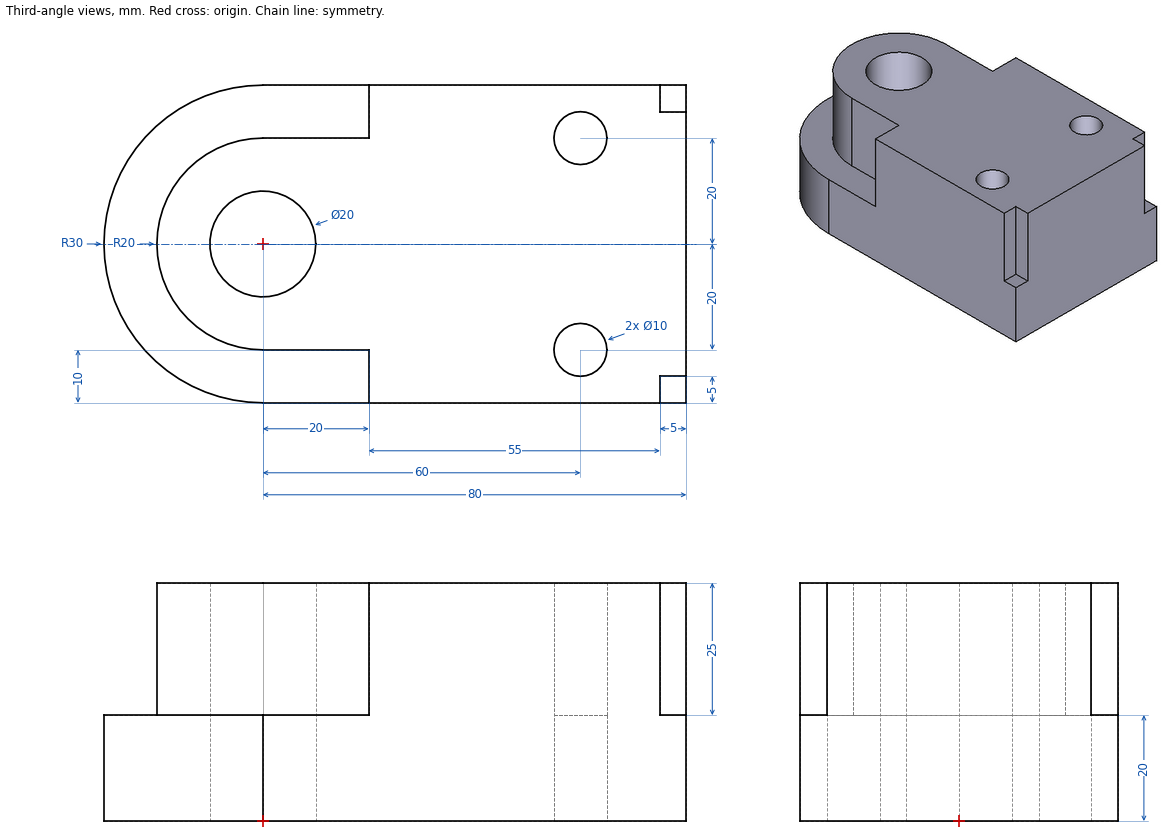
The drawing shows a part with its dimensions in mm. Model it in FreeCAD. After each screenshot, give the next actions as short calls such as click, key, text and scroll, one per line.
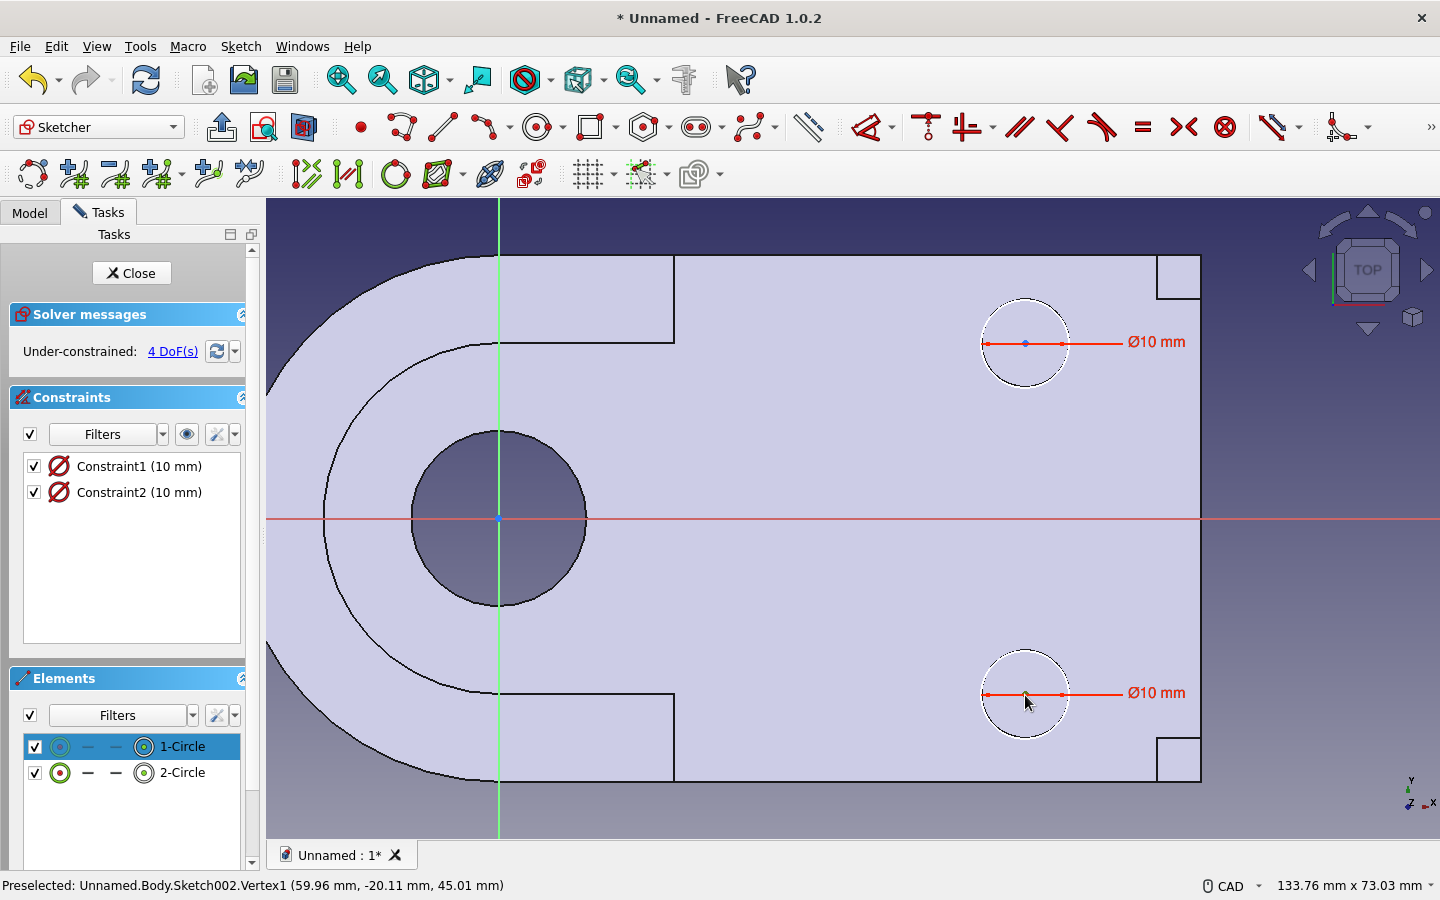
click(1025, 344)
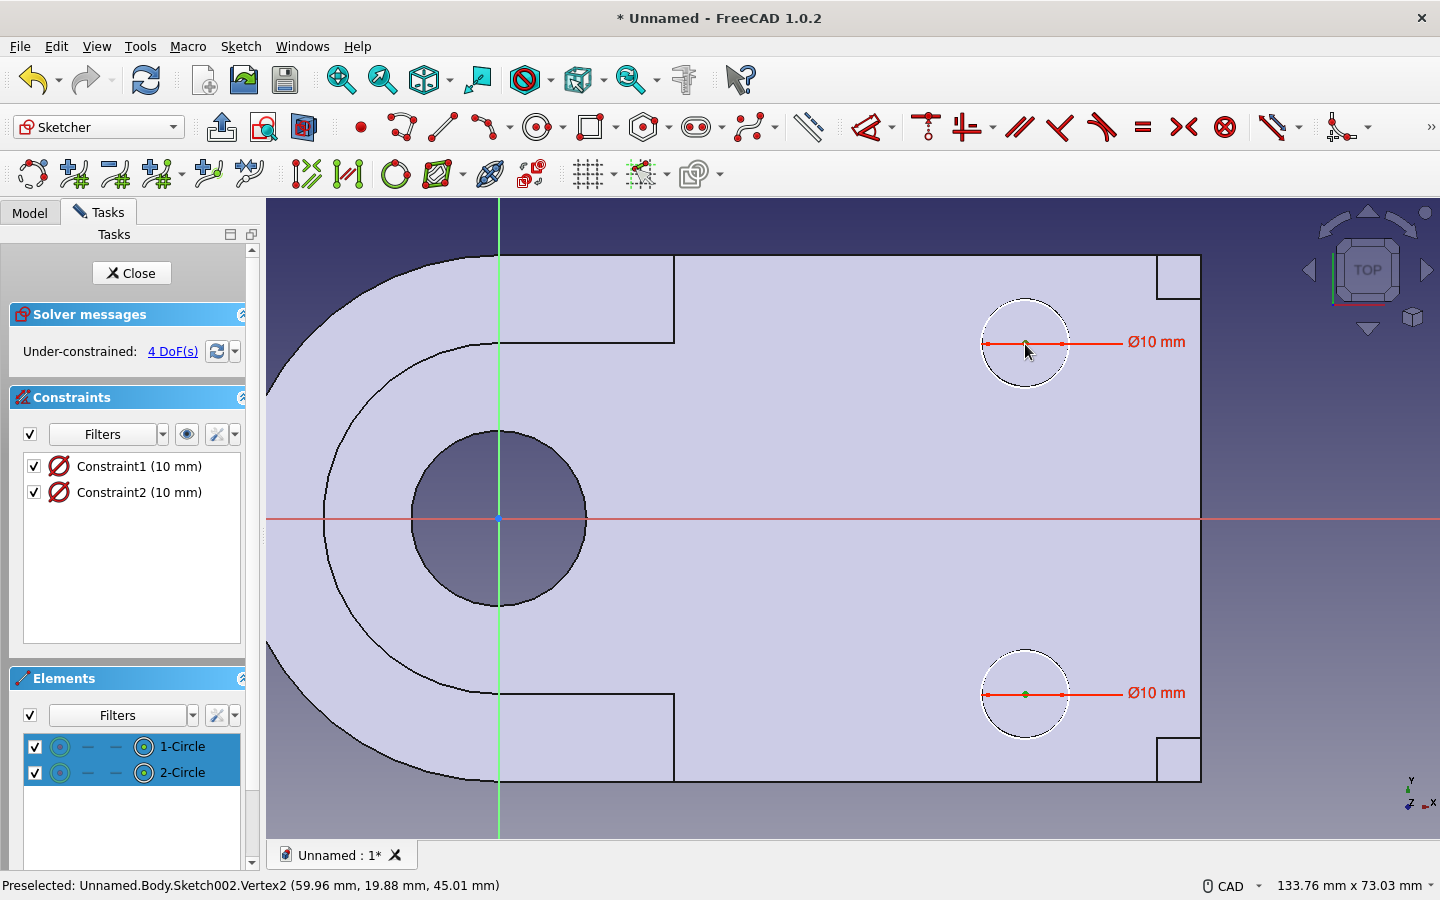
click(992, 128)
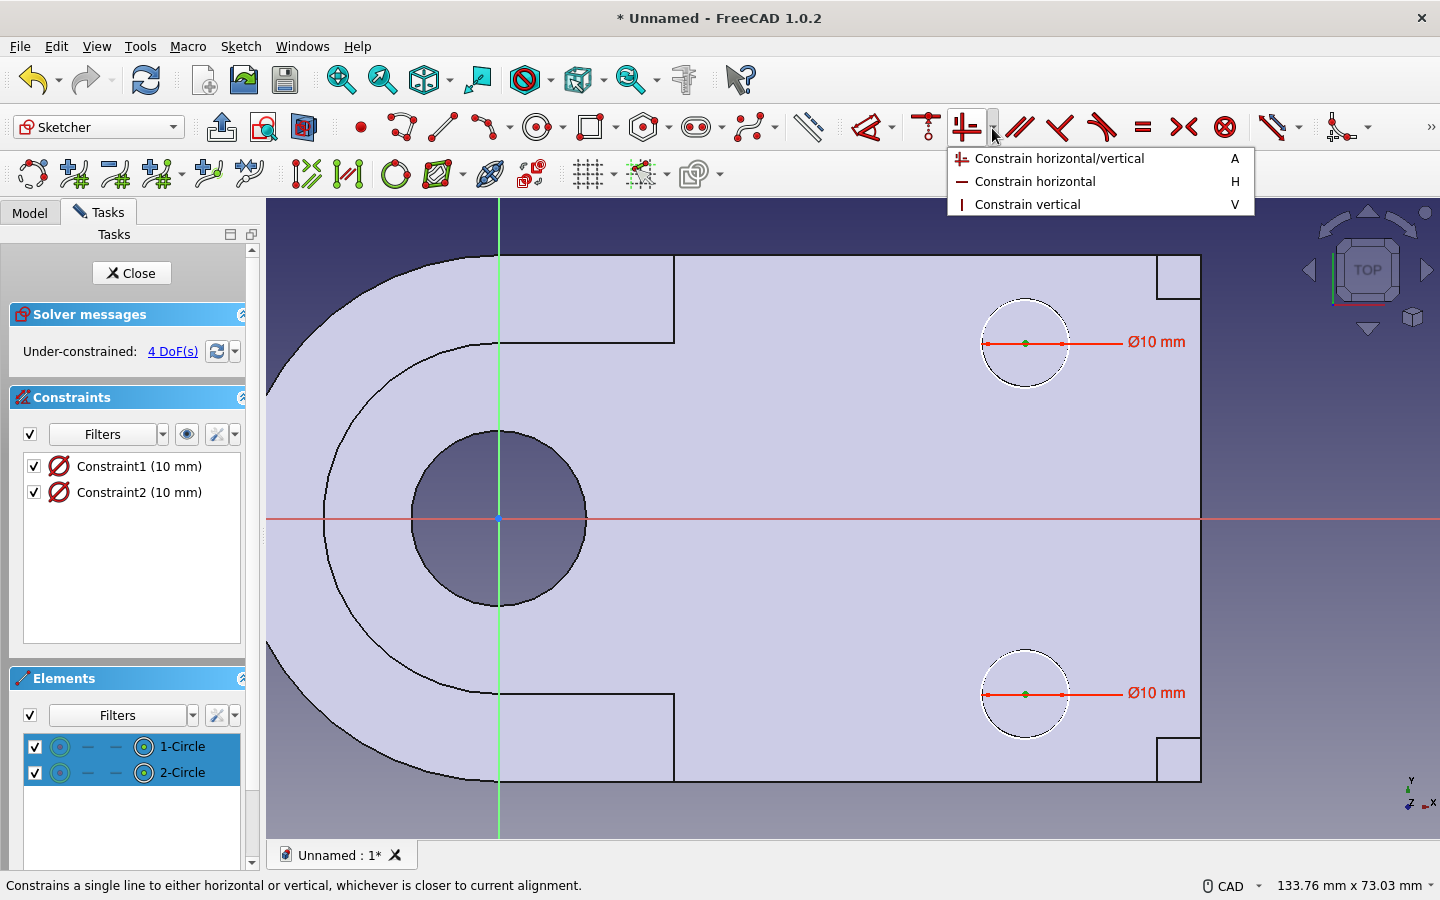
click(1101, 204)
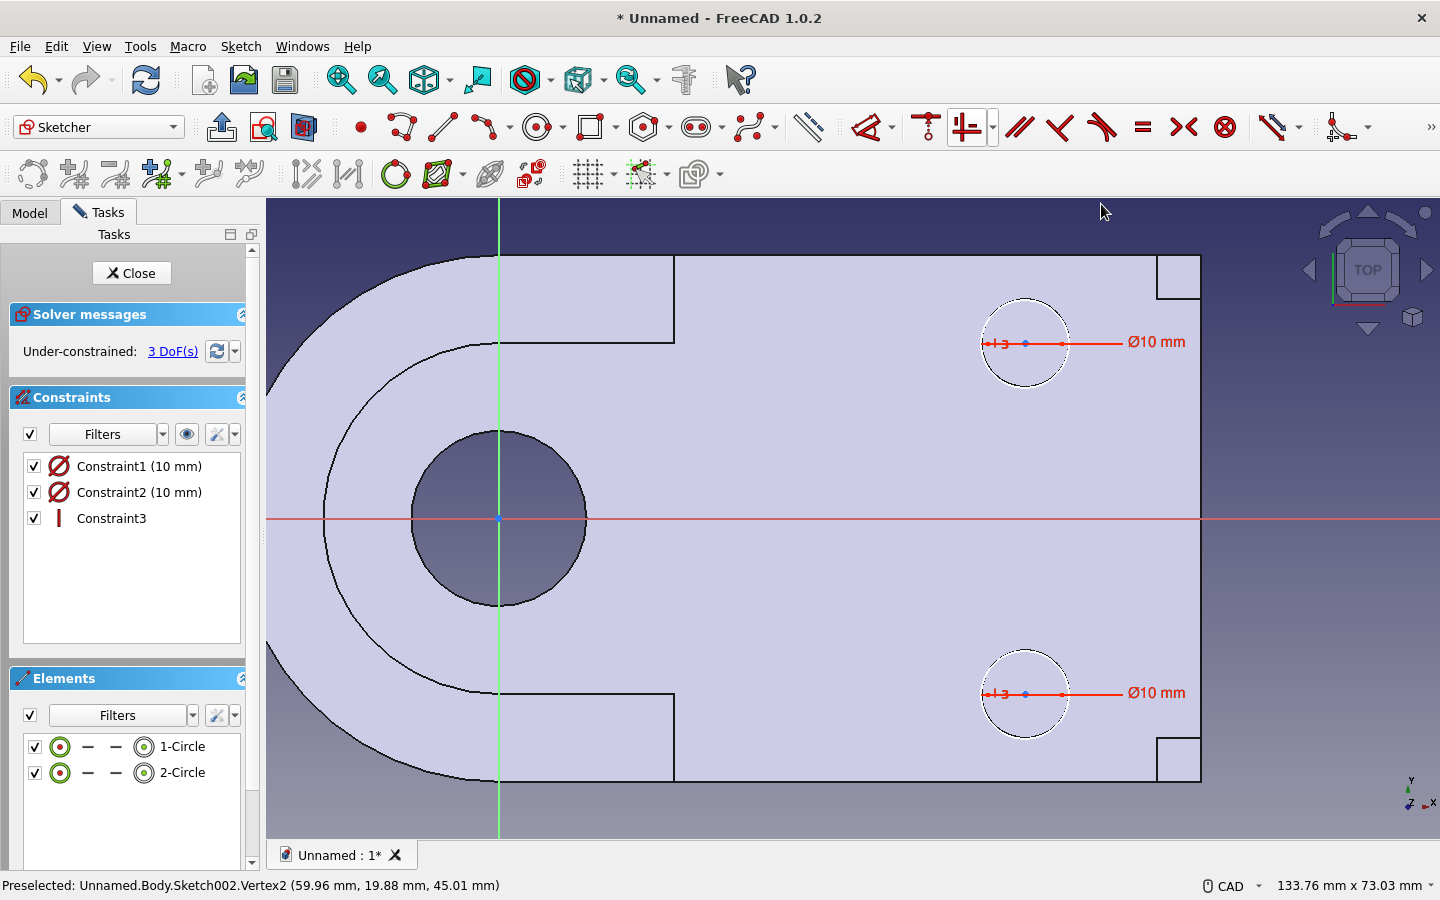
click(866, 128)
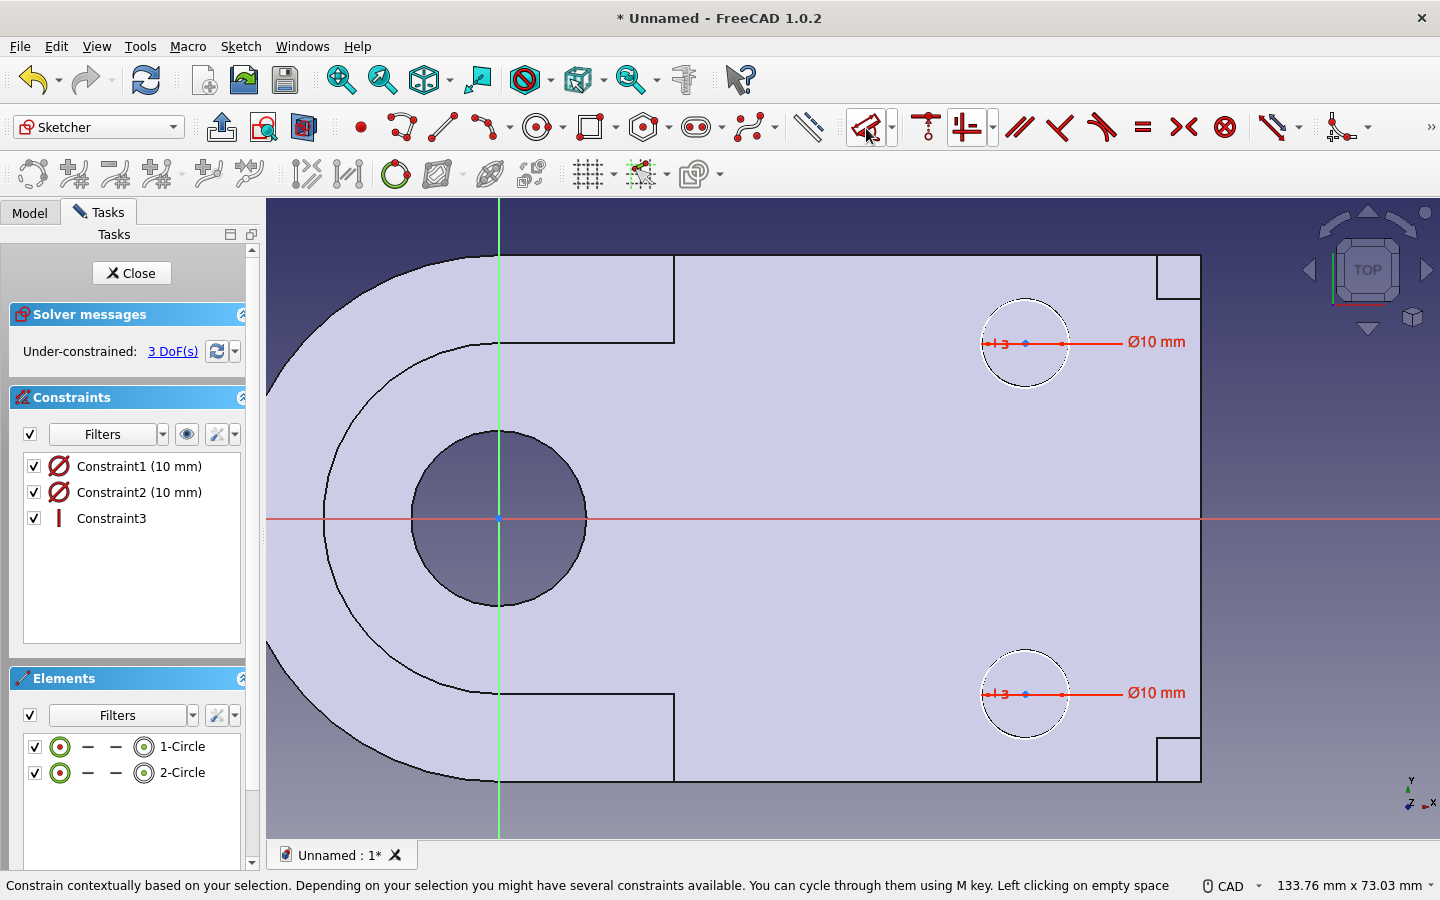
click(1025, 695)
click(762, 729)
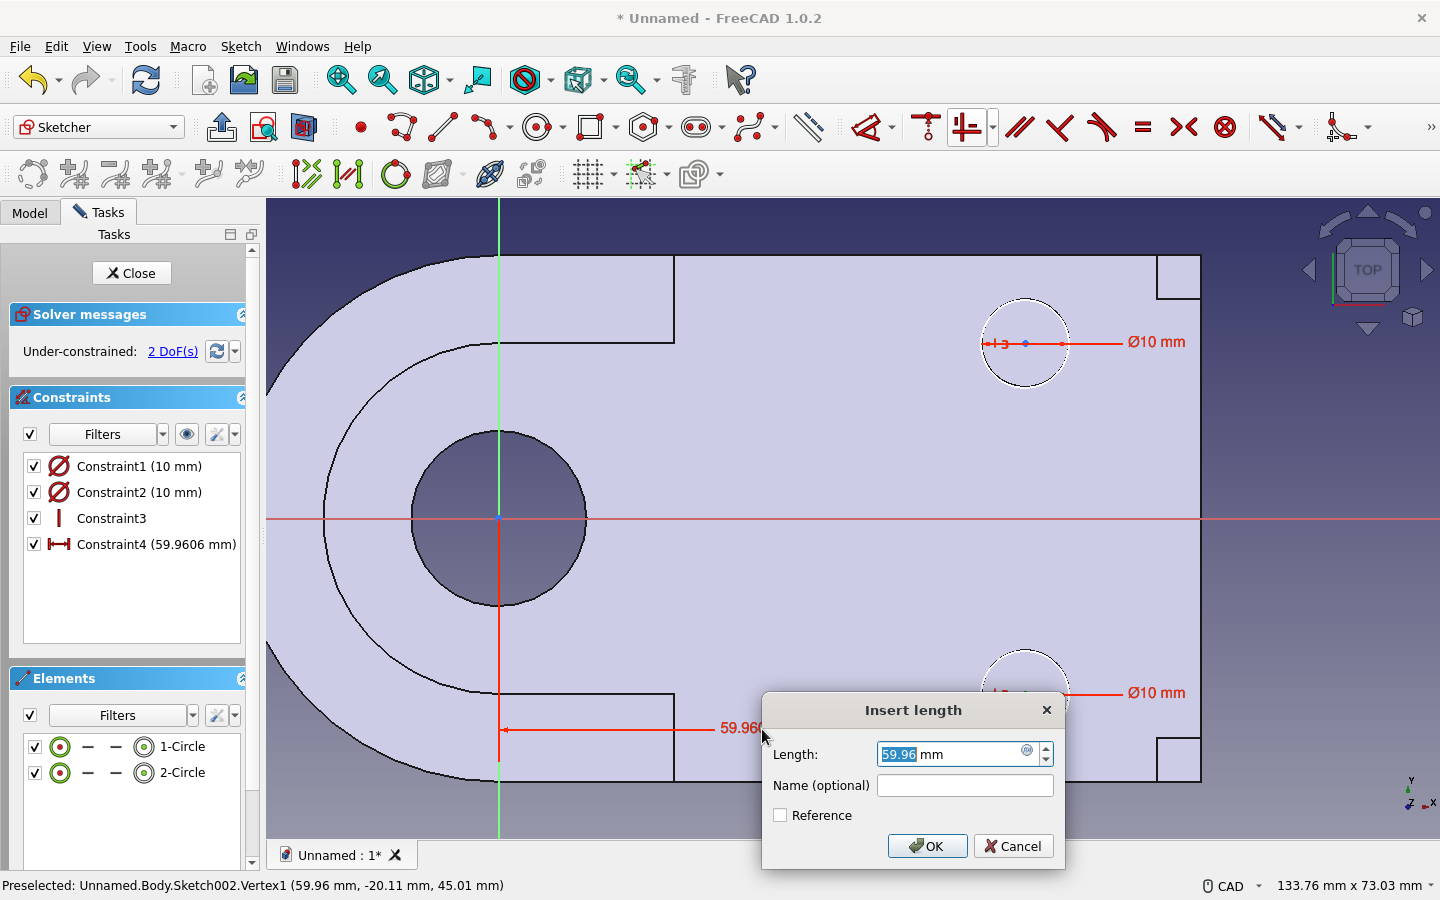
text(60)
key(Return)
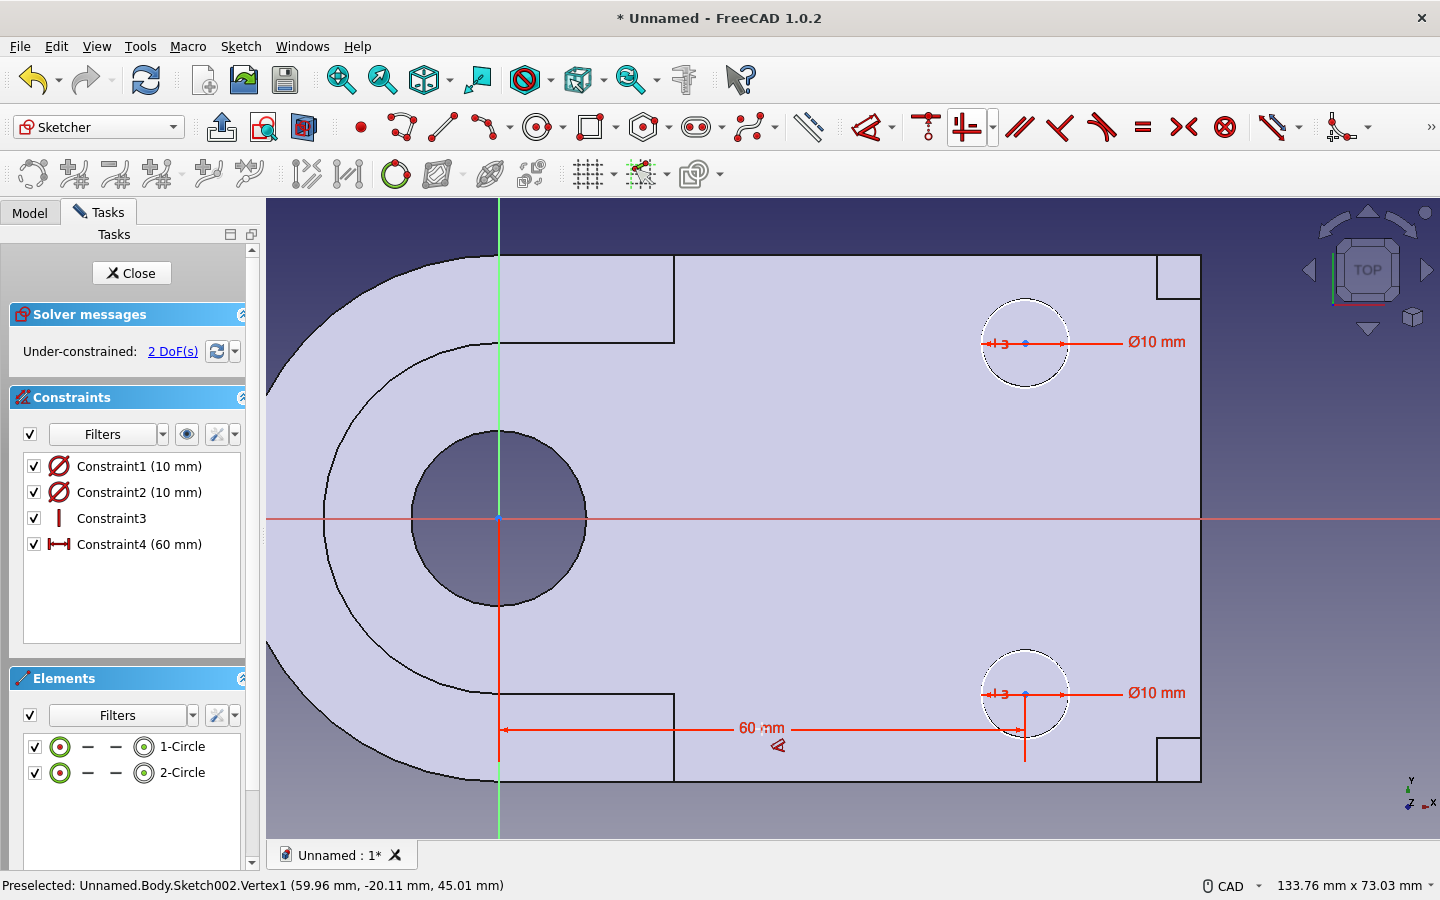
click(1025, 695)
click(465, 607)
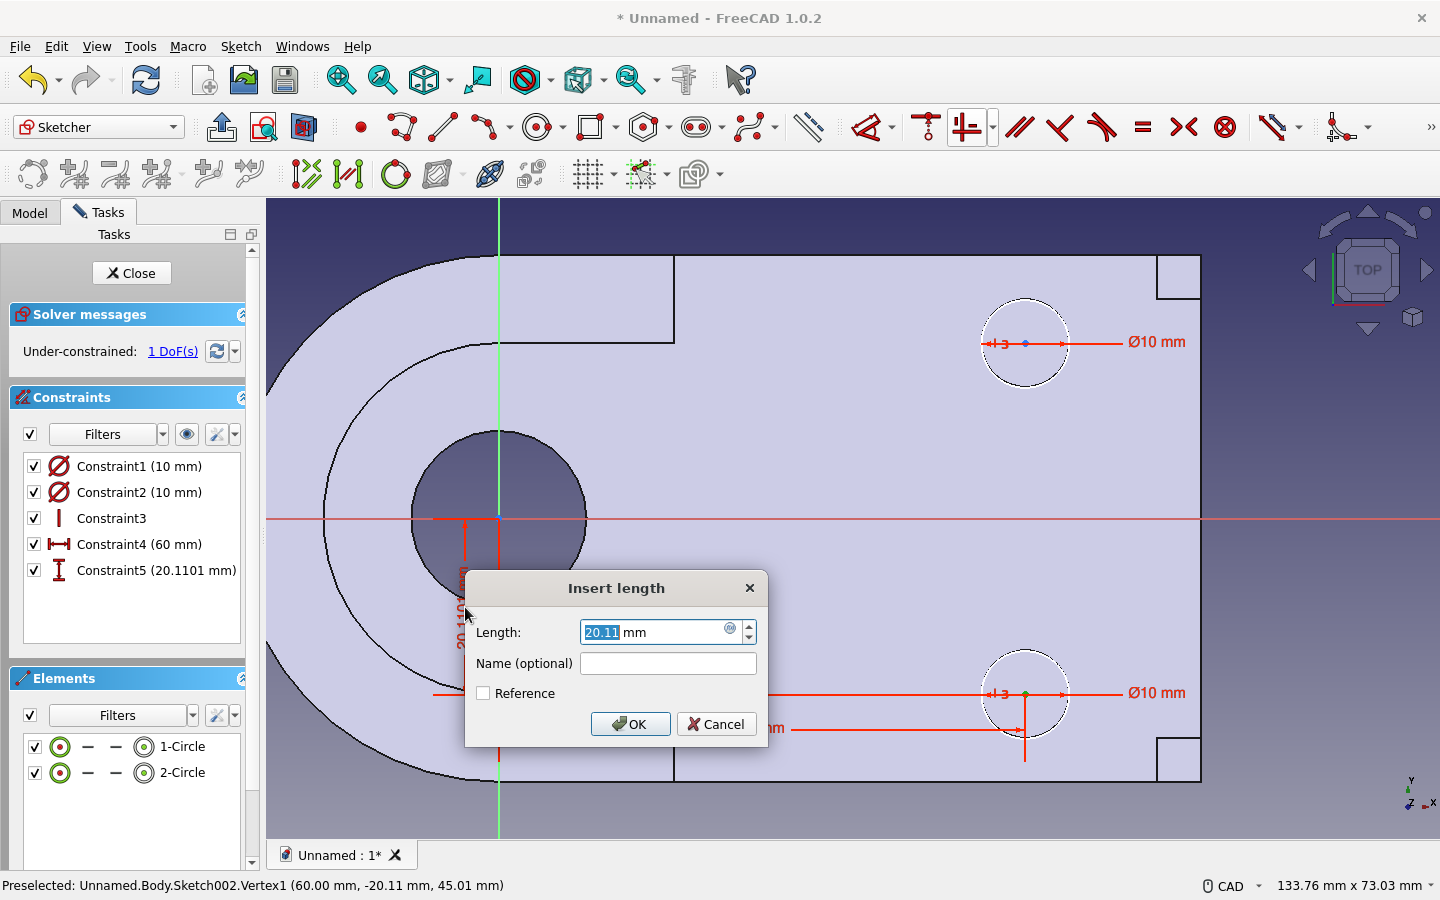
text(20)
key(Return)